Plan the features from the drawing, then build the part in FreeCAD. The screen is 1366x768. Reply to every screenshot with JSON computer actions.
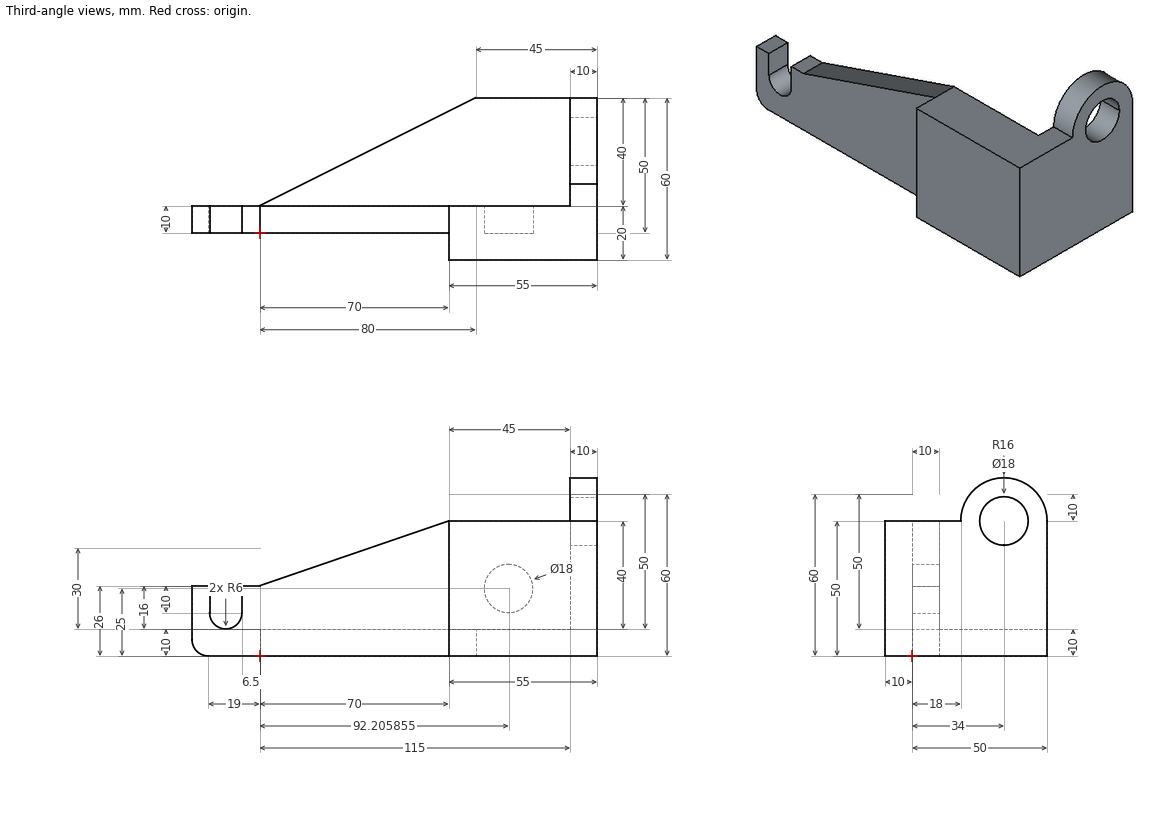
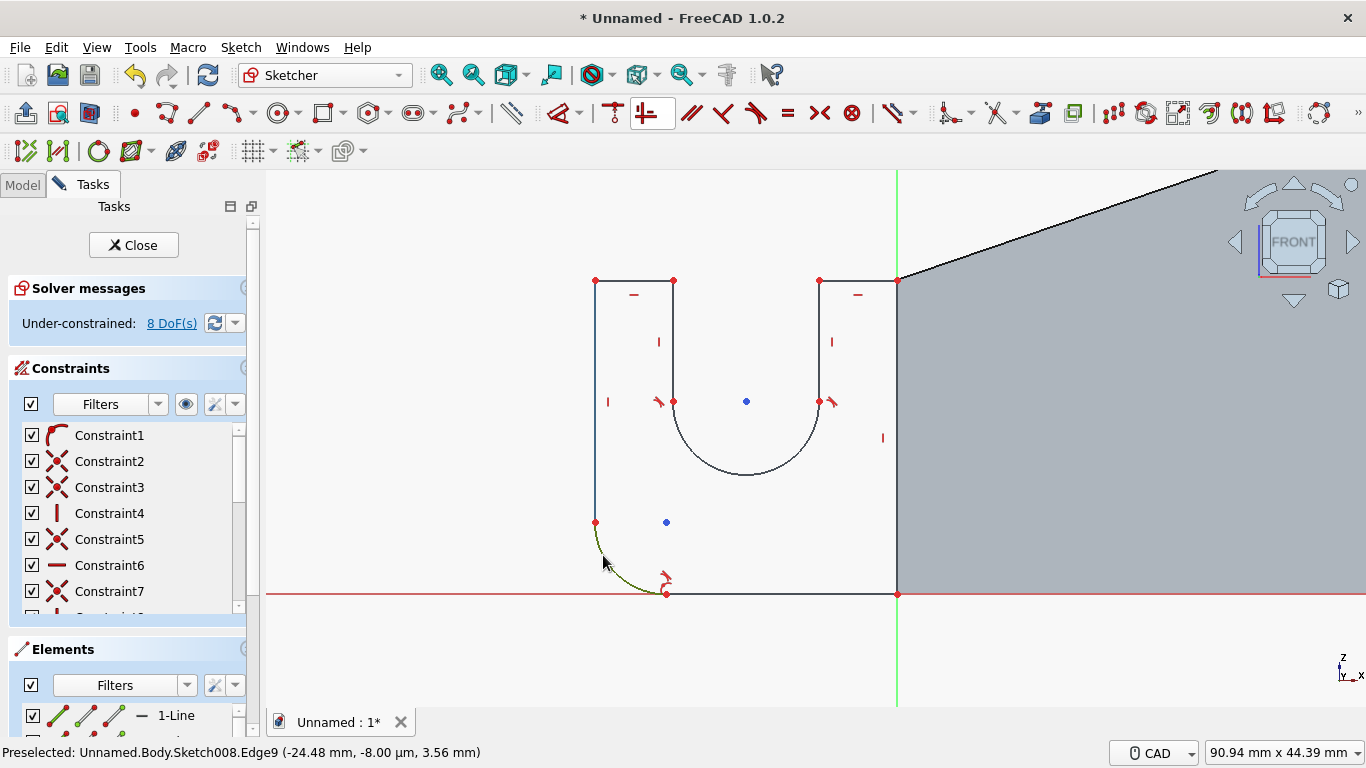
{"action": "left_click", "coordinate": [756, 114]}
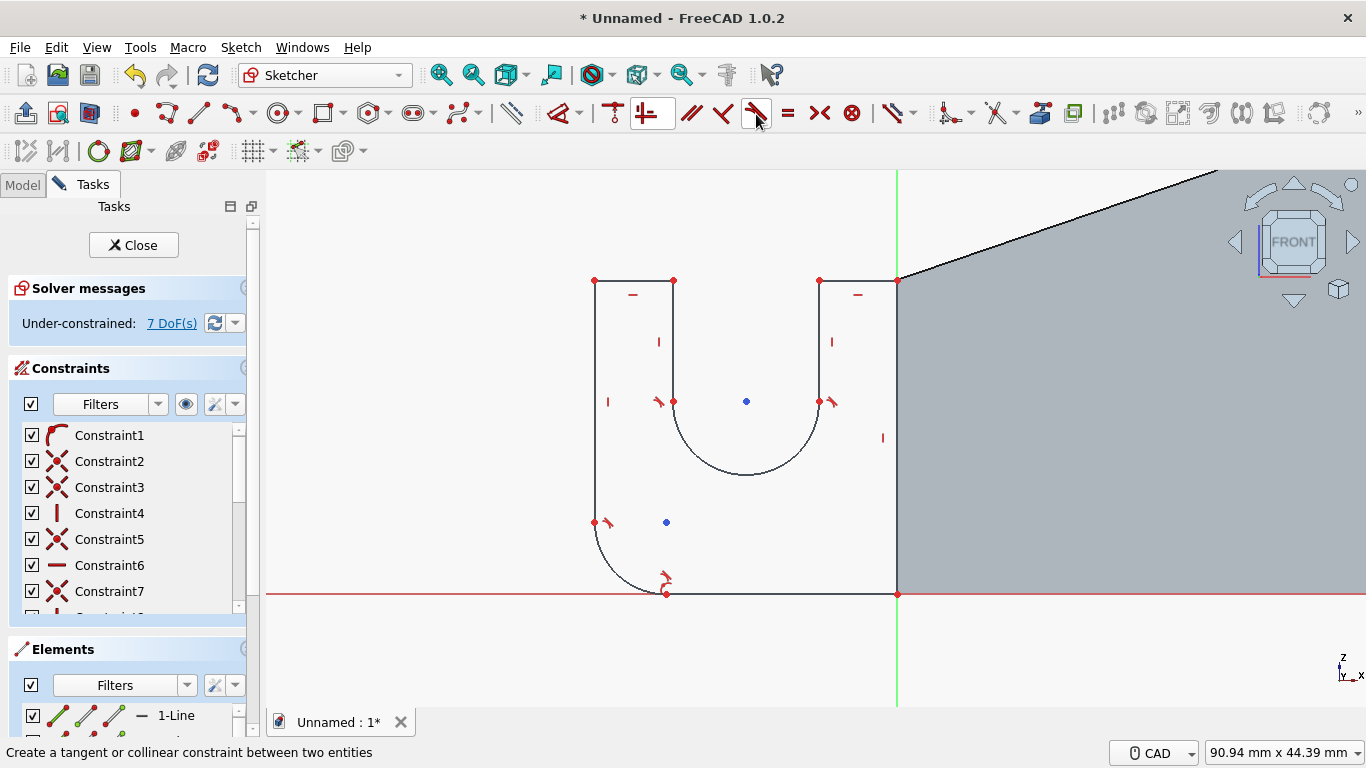
{"action": "left_click", "coordinate": [703, 461]}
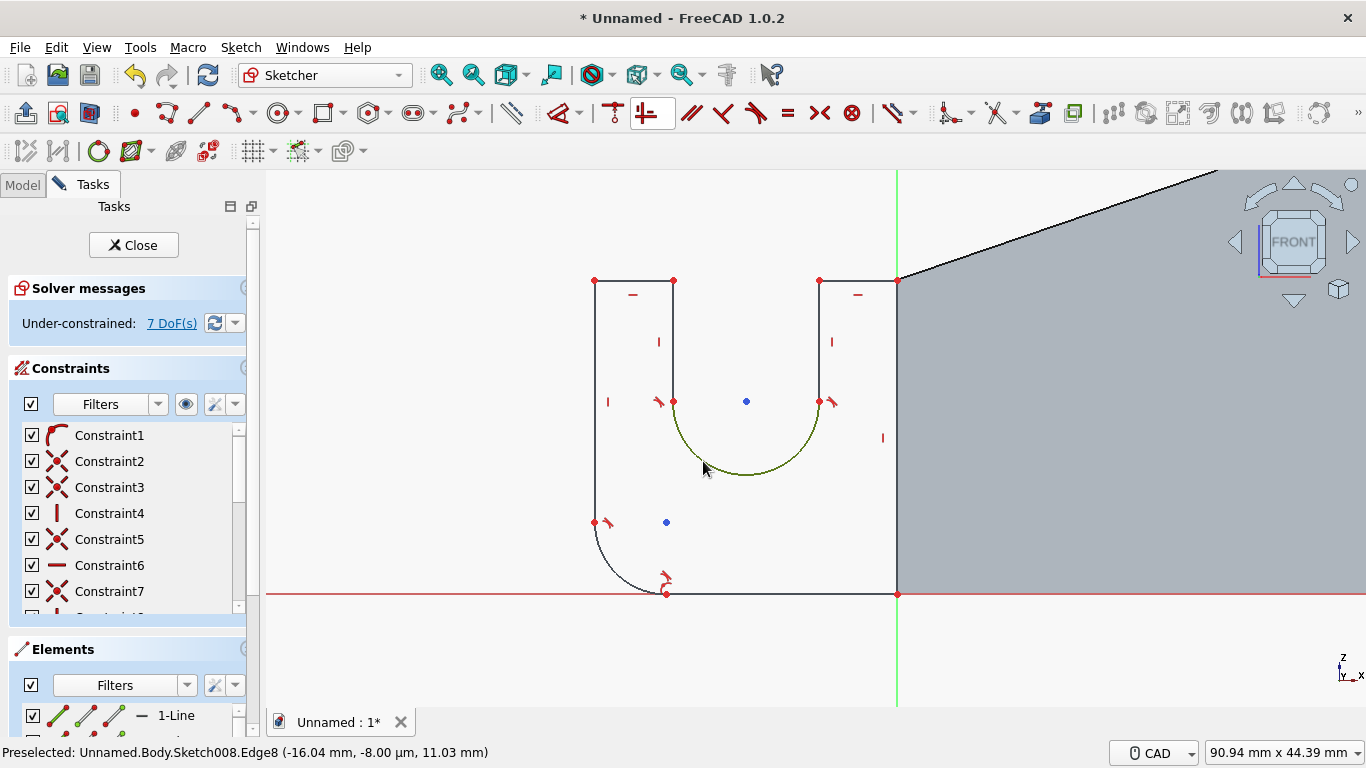
{"action": "left_click", "coordinate": [603, 555]}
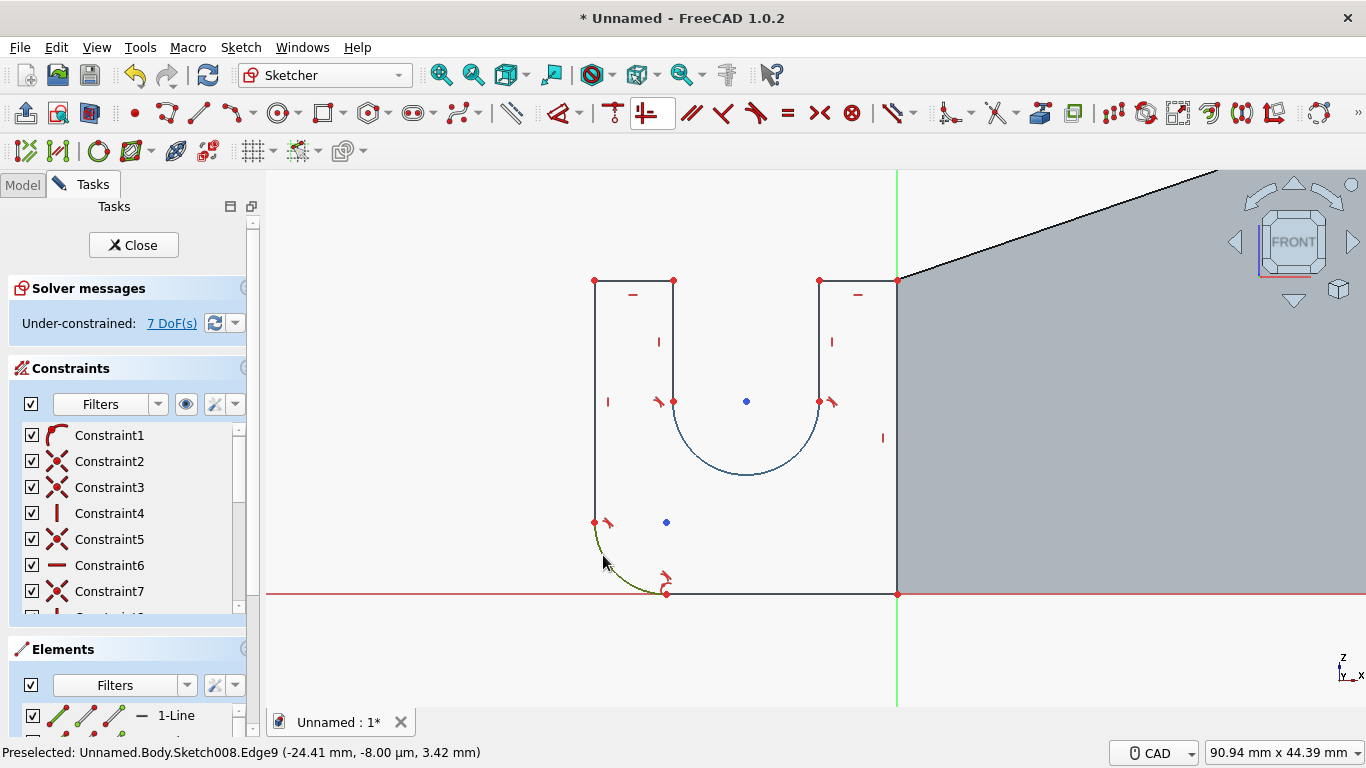
{"action": "left_click", "coordinate": [788, 114]}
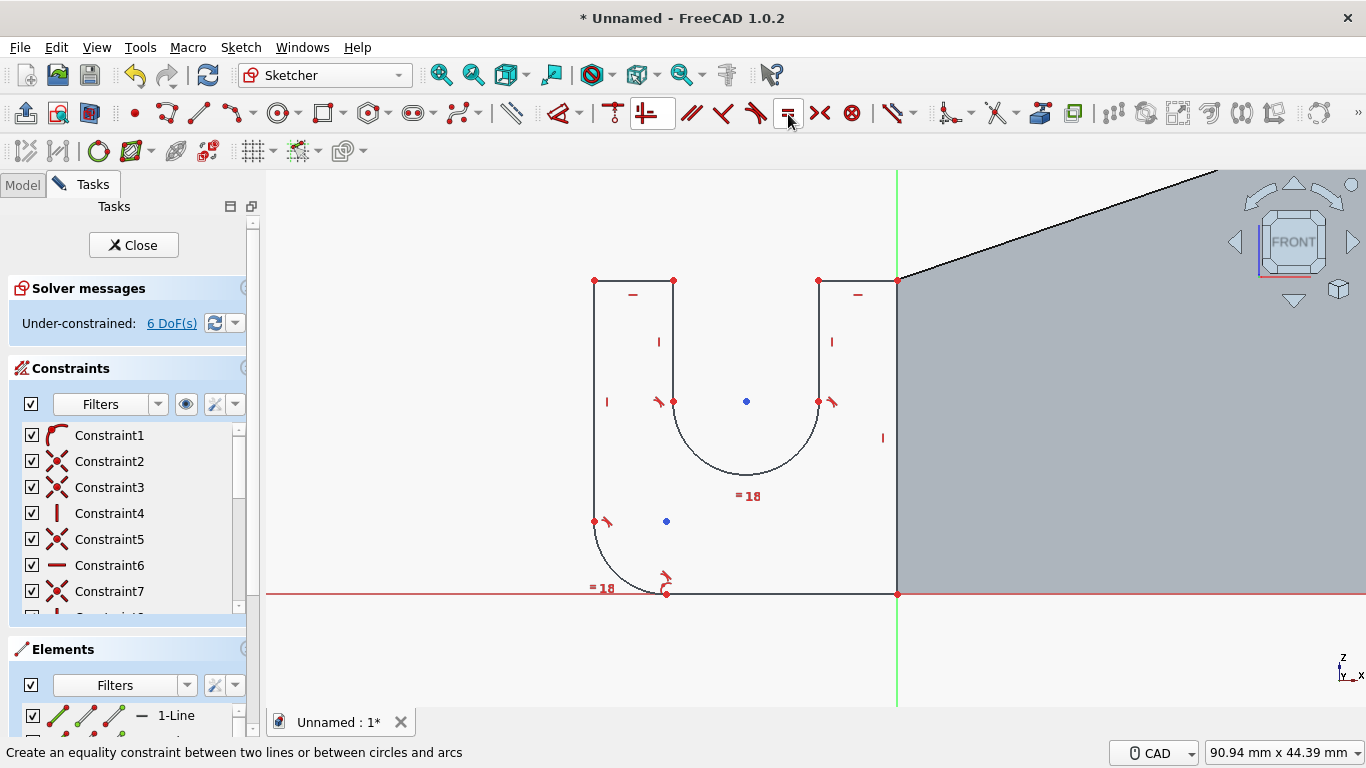
{"action": "left_click", "coordinate": [558, 114]}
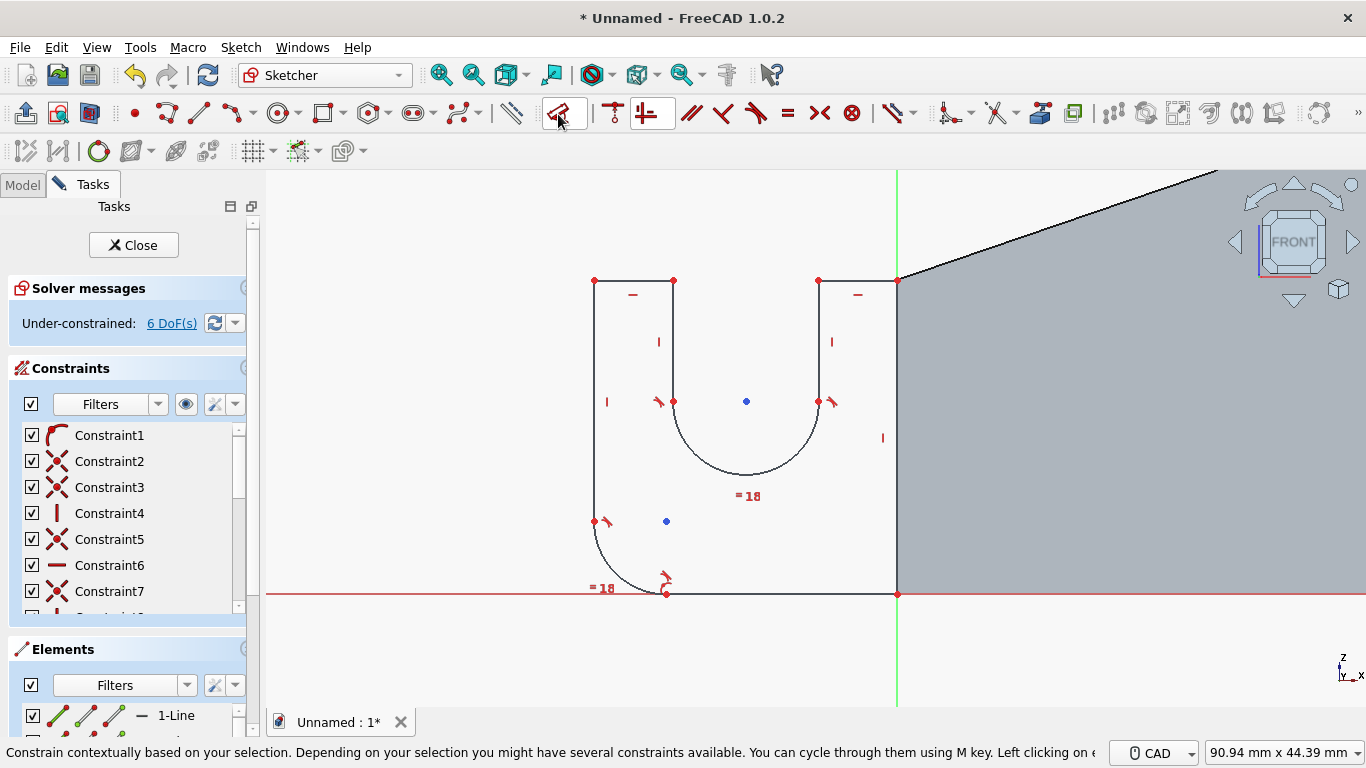
{"action": "left_click", "coordinate": [703, 461]}
{"action": "left_click", "coordinate": [684, 487]}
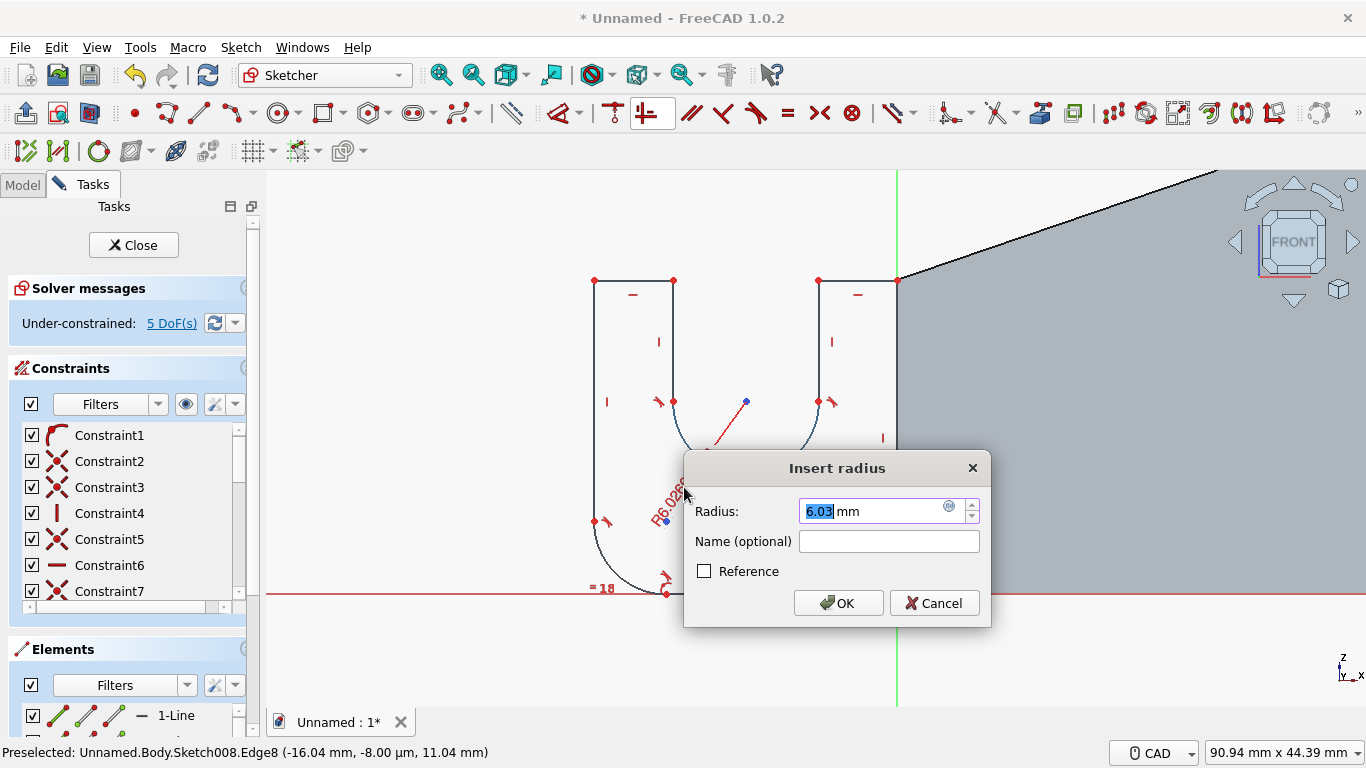
{"action": "type", "text": "6"}
{"action": "key", "text": "Return"}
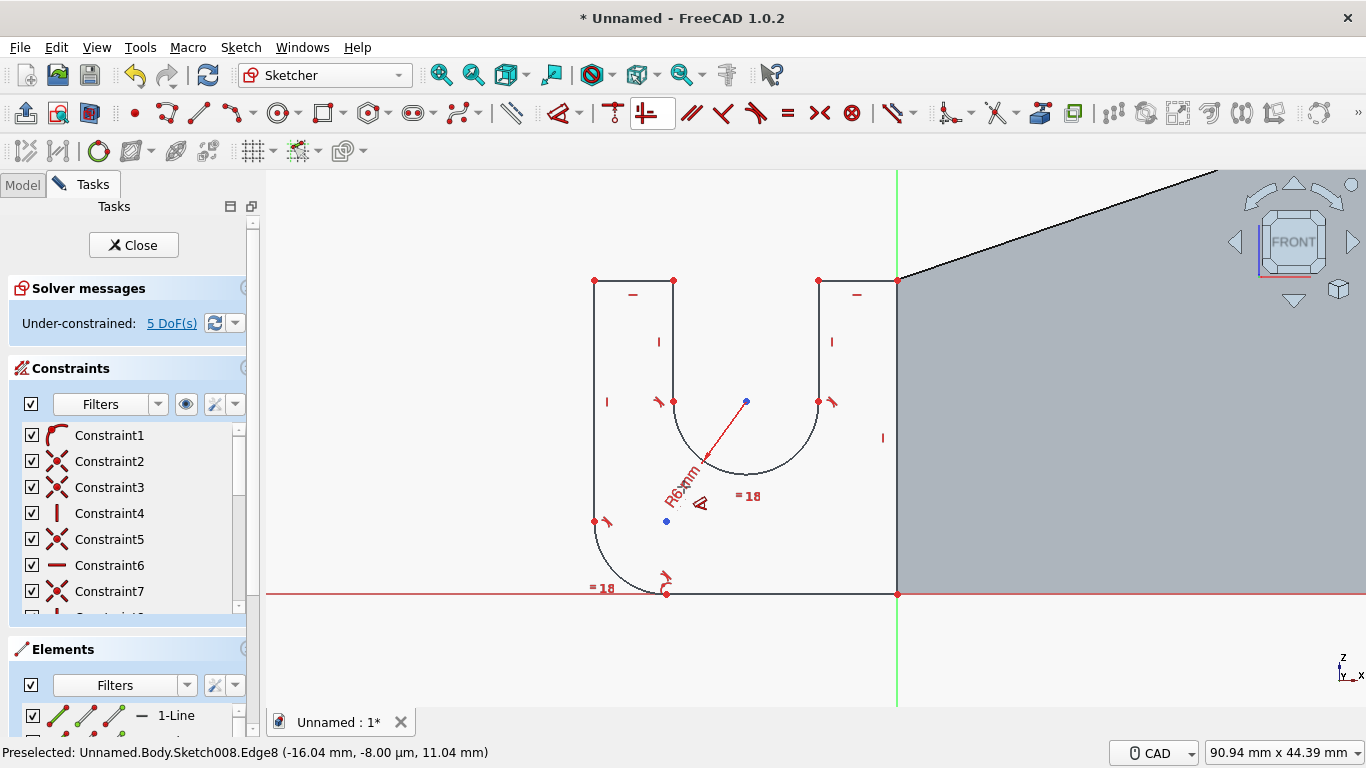
{"action": "left_click", "coordinate": [736, 594]}
{"action": "left_click", "coordinate": [782, 628]}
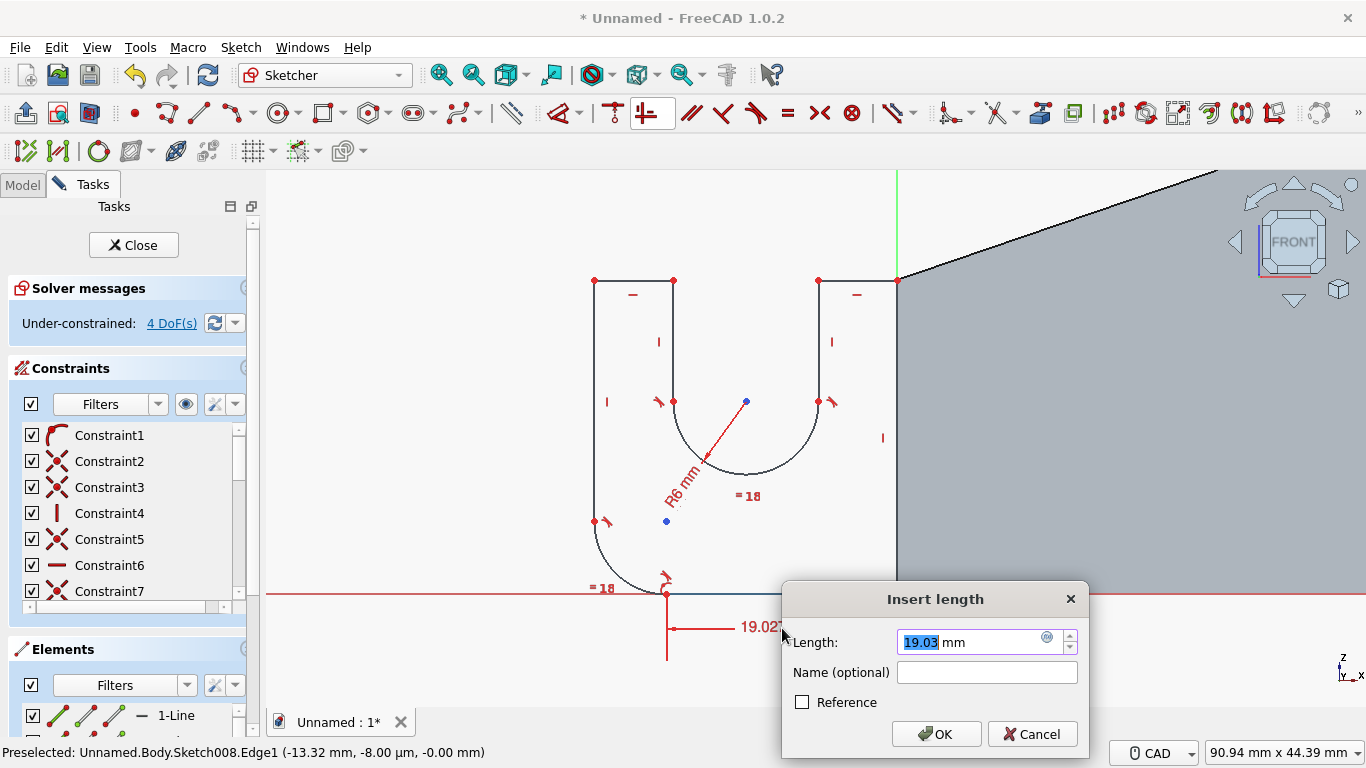
{"action": "type", "text": "19"}
{"action": "key", "text": "Return"}